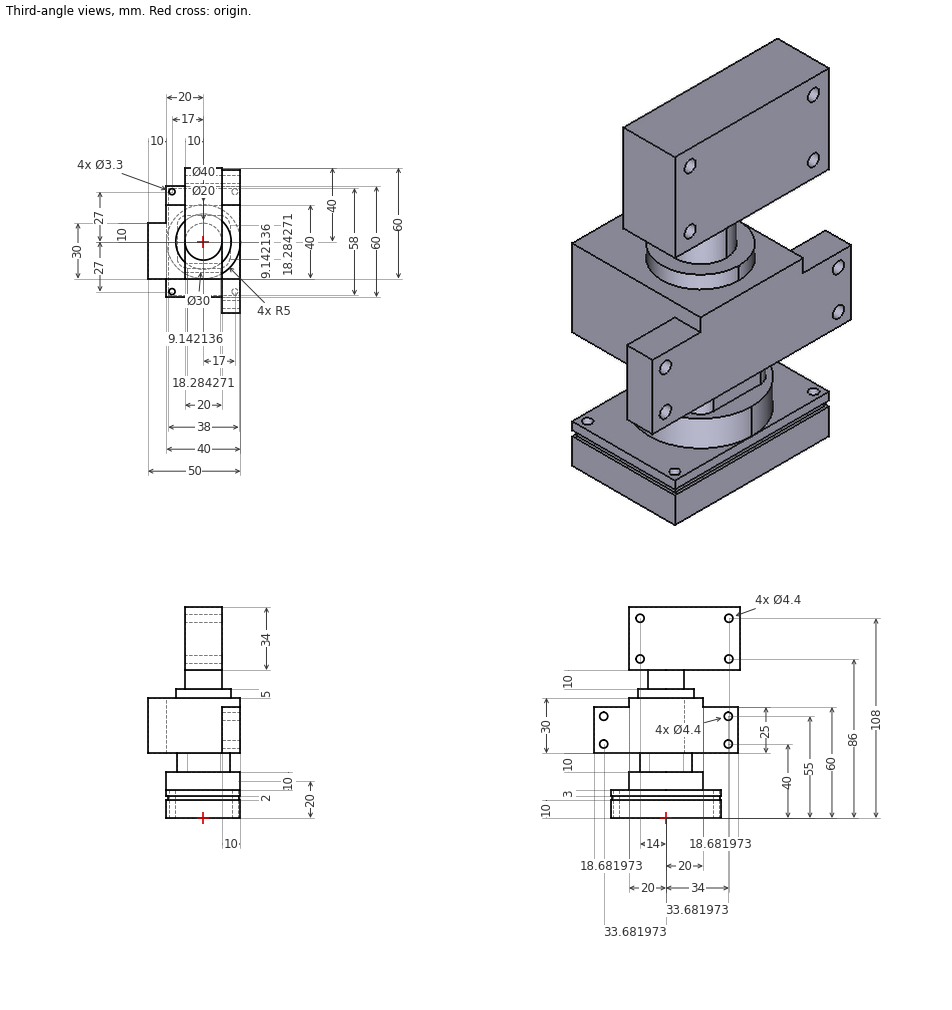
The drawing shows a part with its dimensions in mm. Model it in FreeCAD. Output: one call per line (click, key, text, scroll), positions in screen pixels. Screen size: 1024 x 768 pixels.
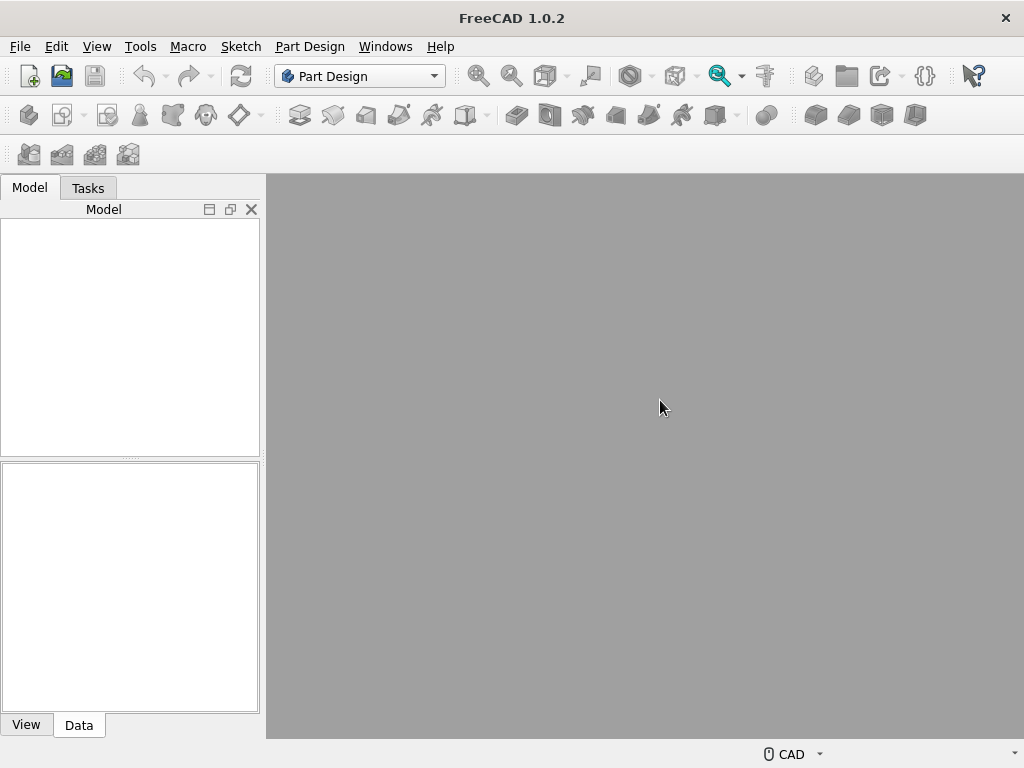
key(ctrl+n)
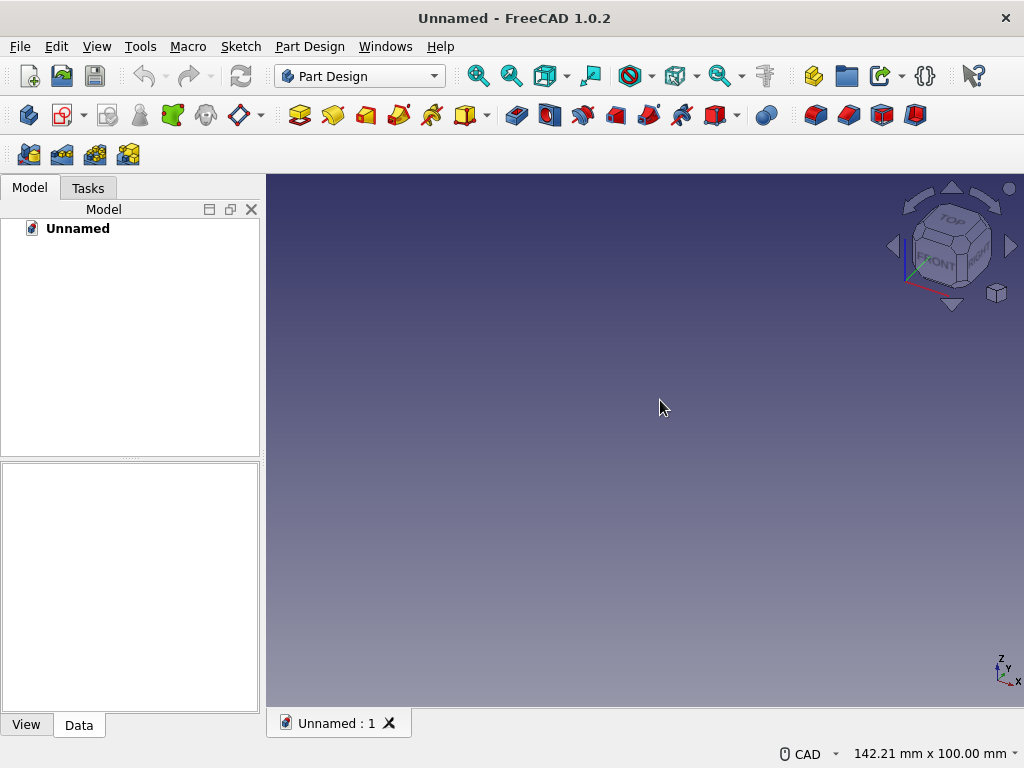
click(62, 116)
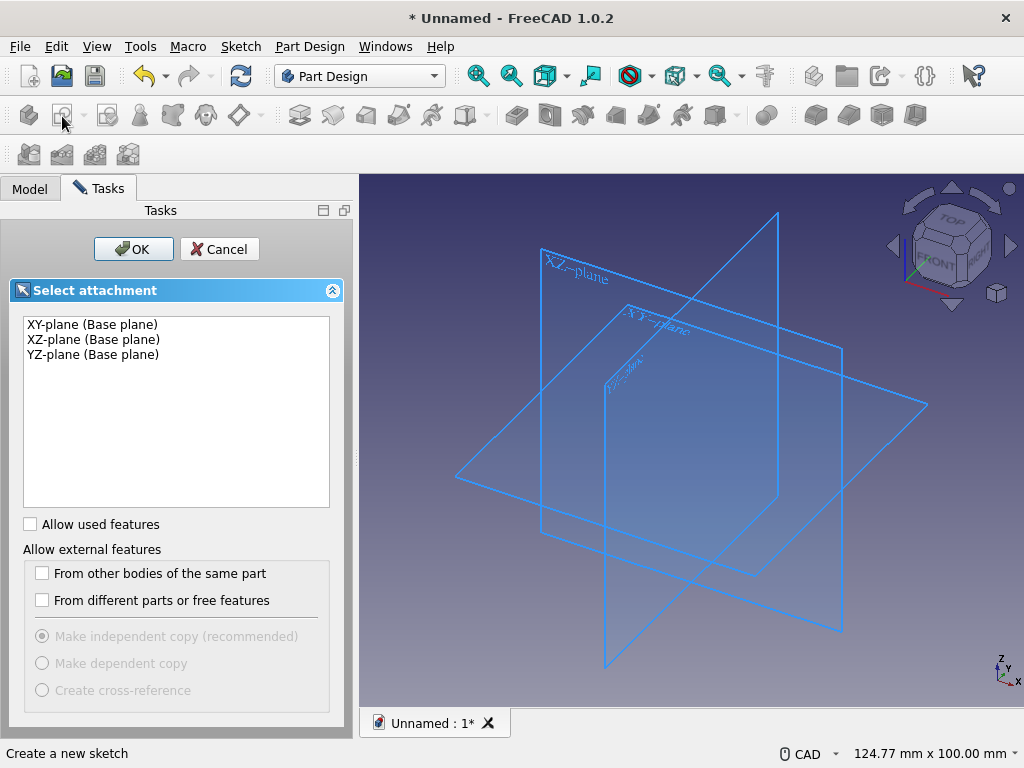
click(84, 324)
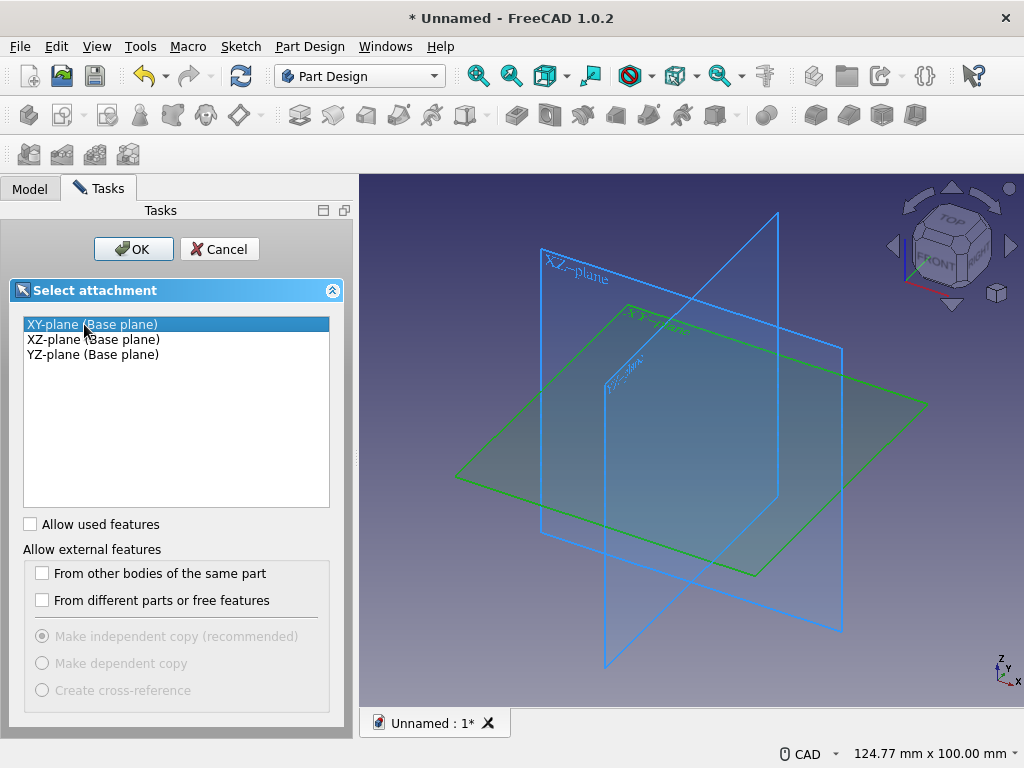
click(134, 249)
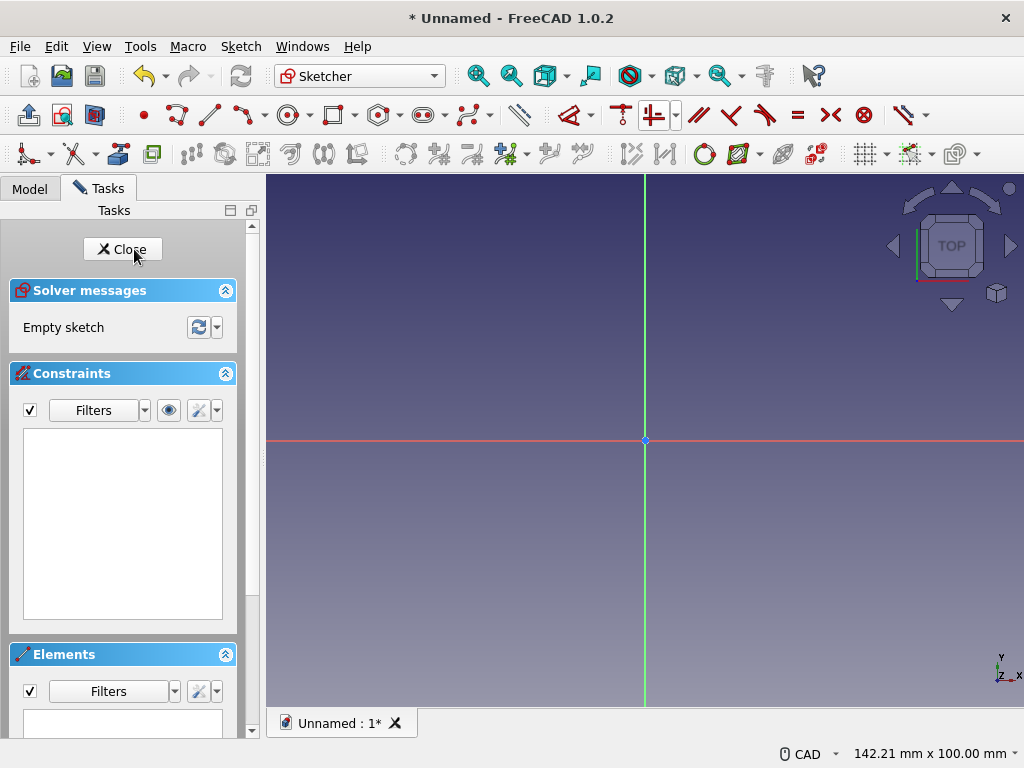
key(g)
key(v)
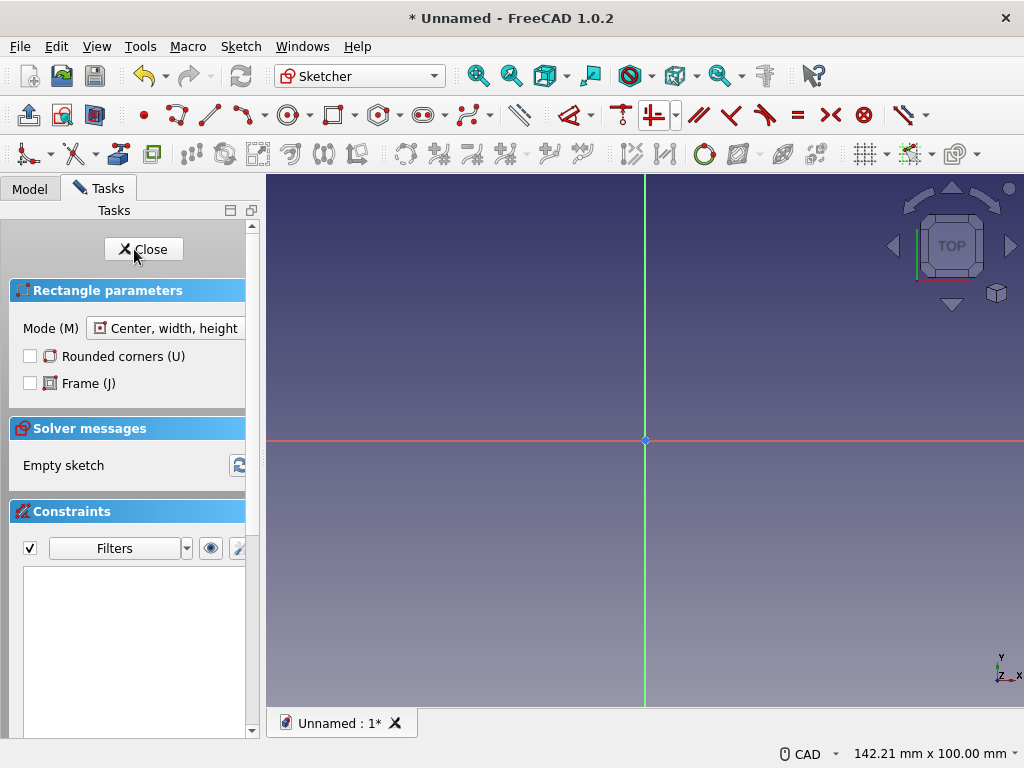
click(645, 440)
move(752, 281)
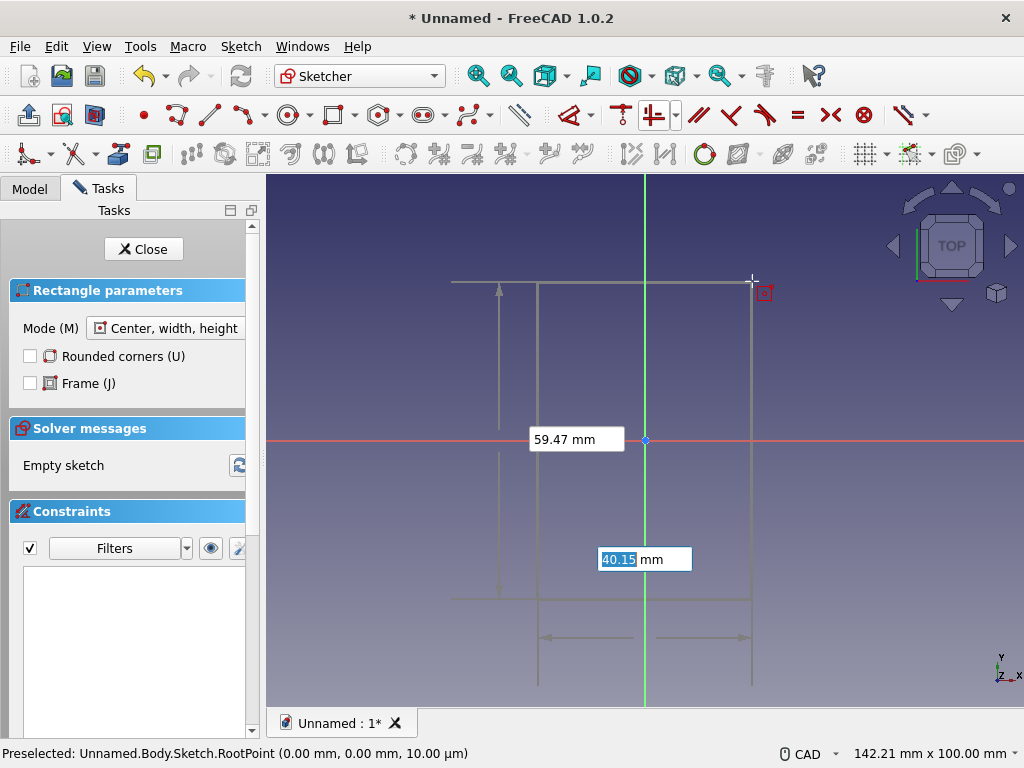
text(40)
key(Tab)
text(60)
key(Return)
key(Escape)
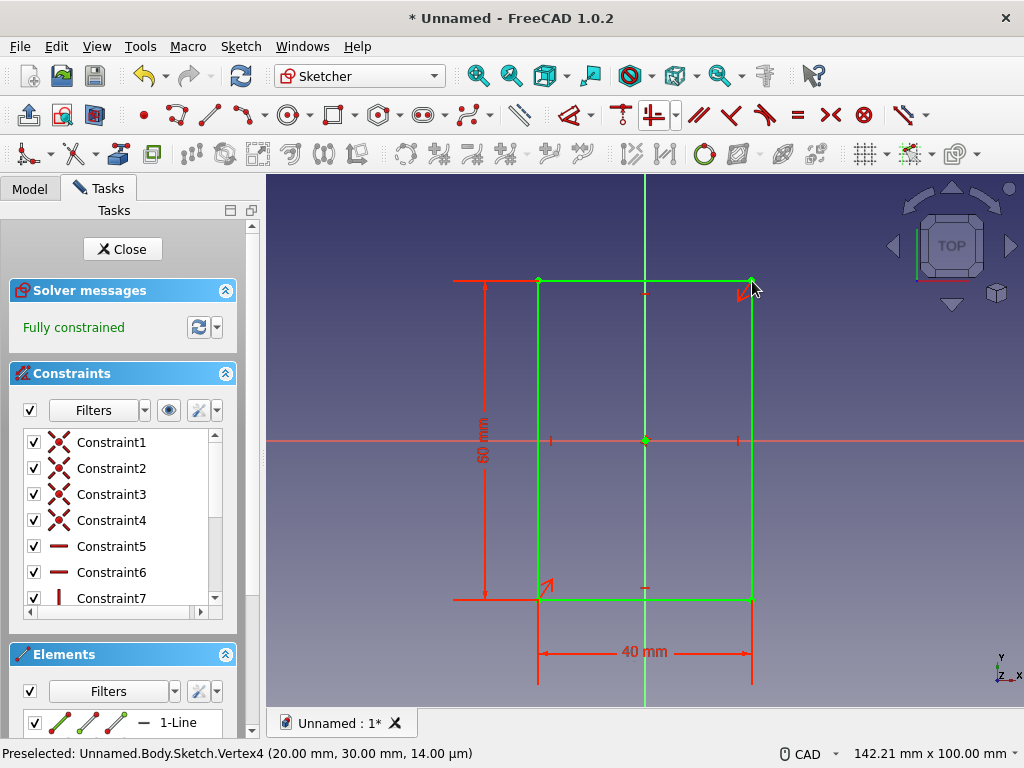
click(123, 249)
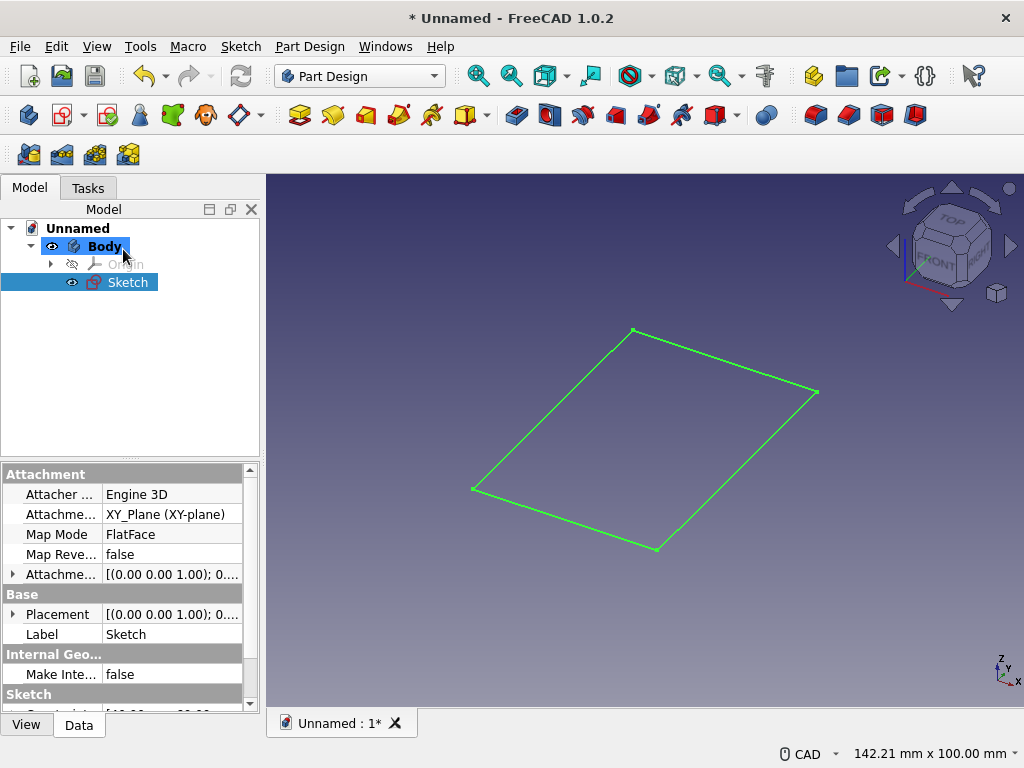
click(300, 116)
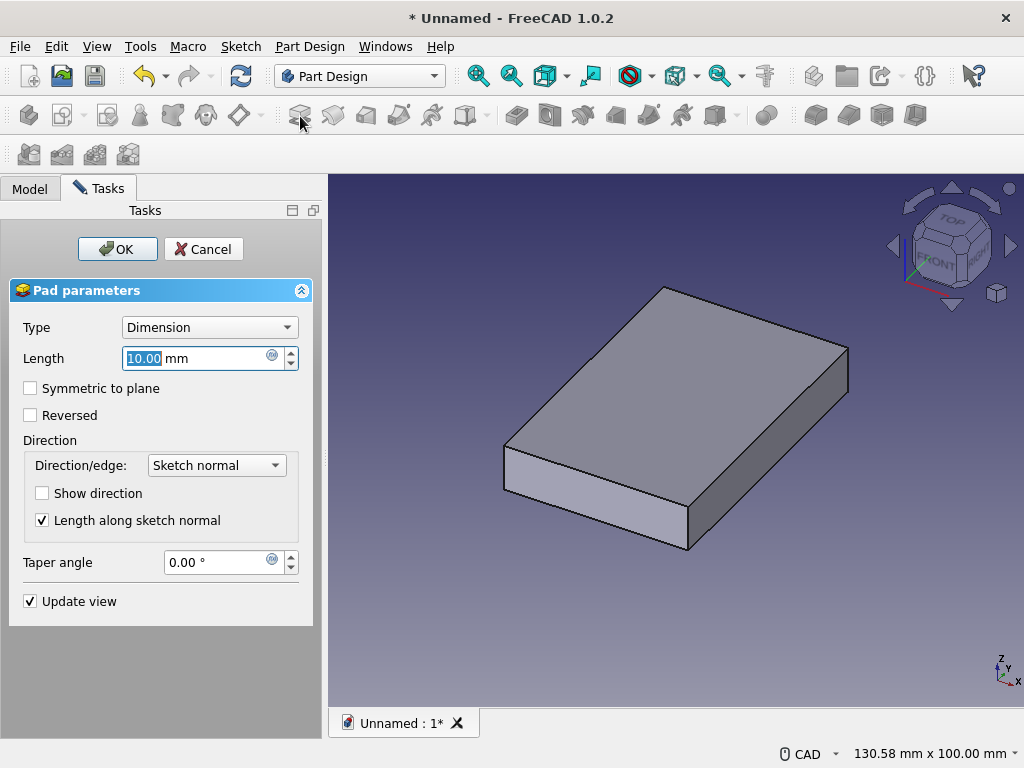
text(10)
key(Tab)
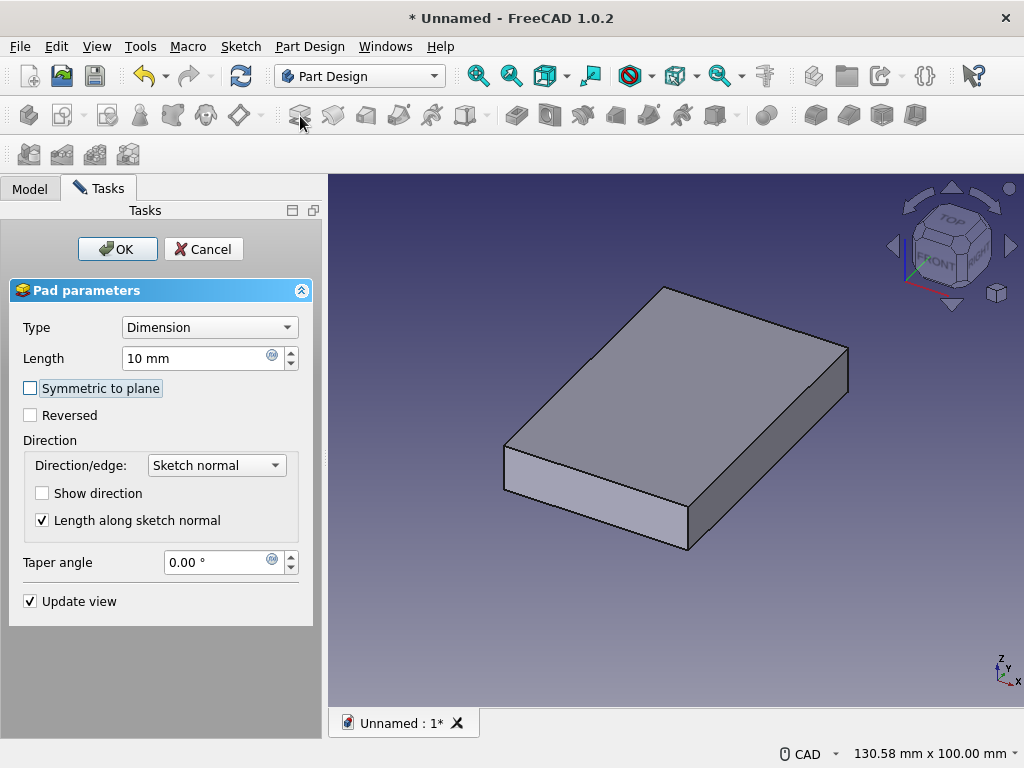
click(118, 249)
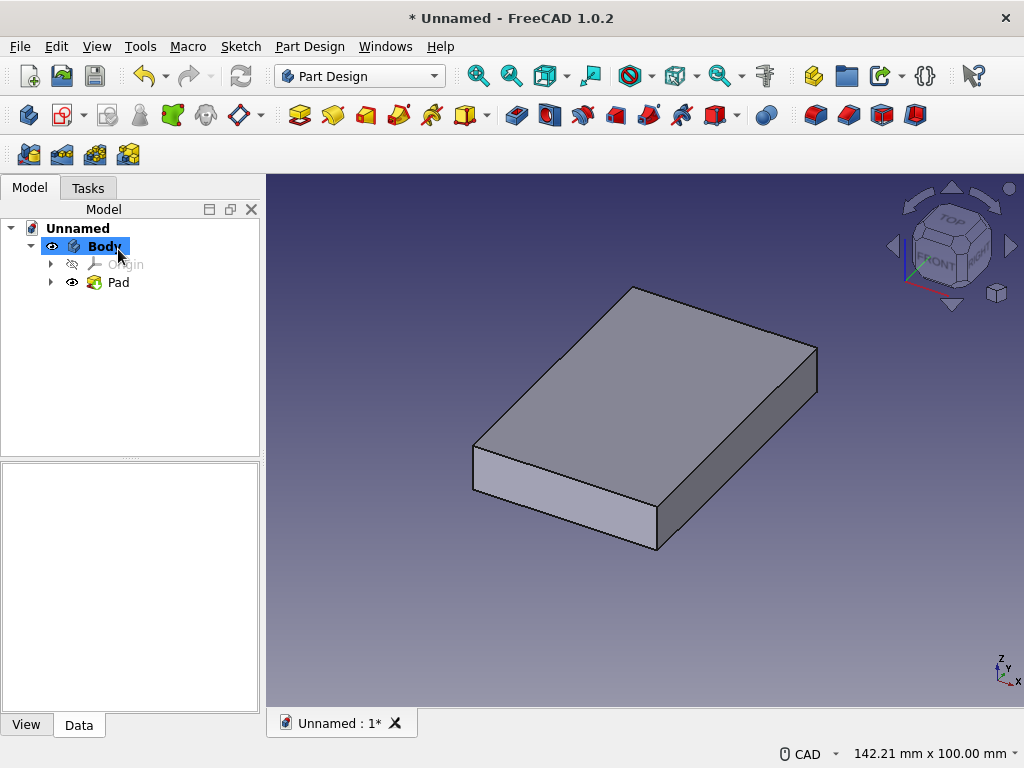
click(668, 373)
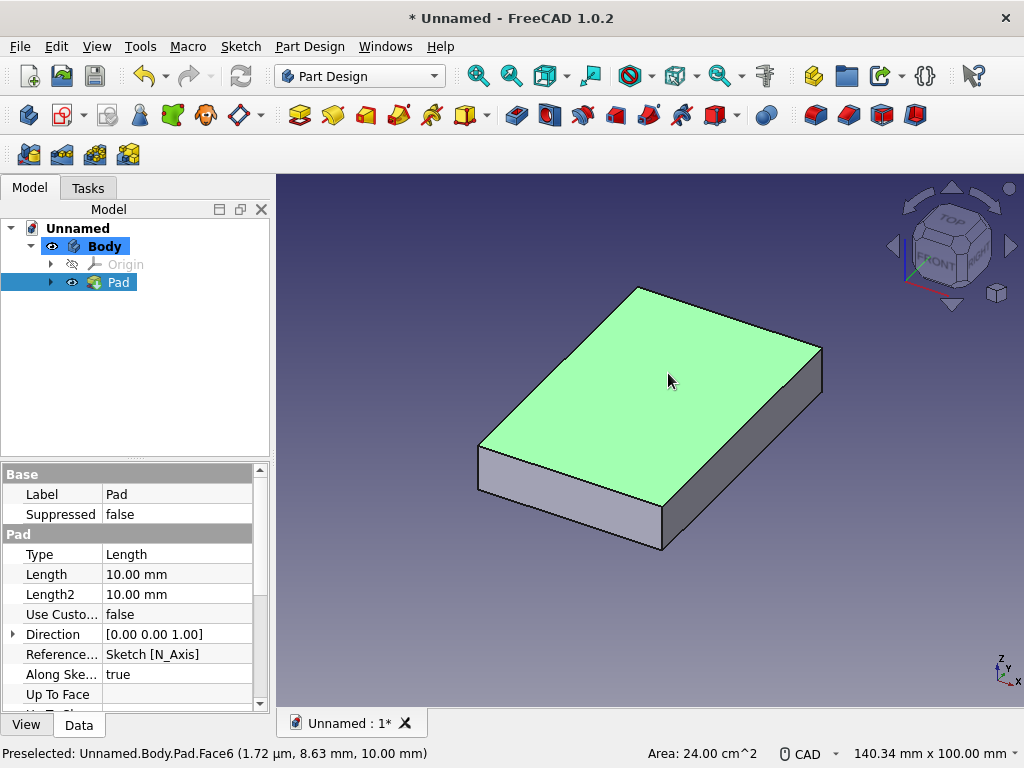
click(62, 116)